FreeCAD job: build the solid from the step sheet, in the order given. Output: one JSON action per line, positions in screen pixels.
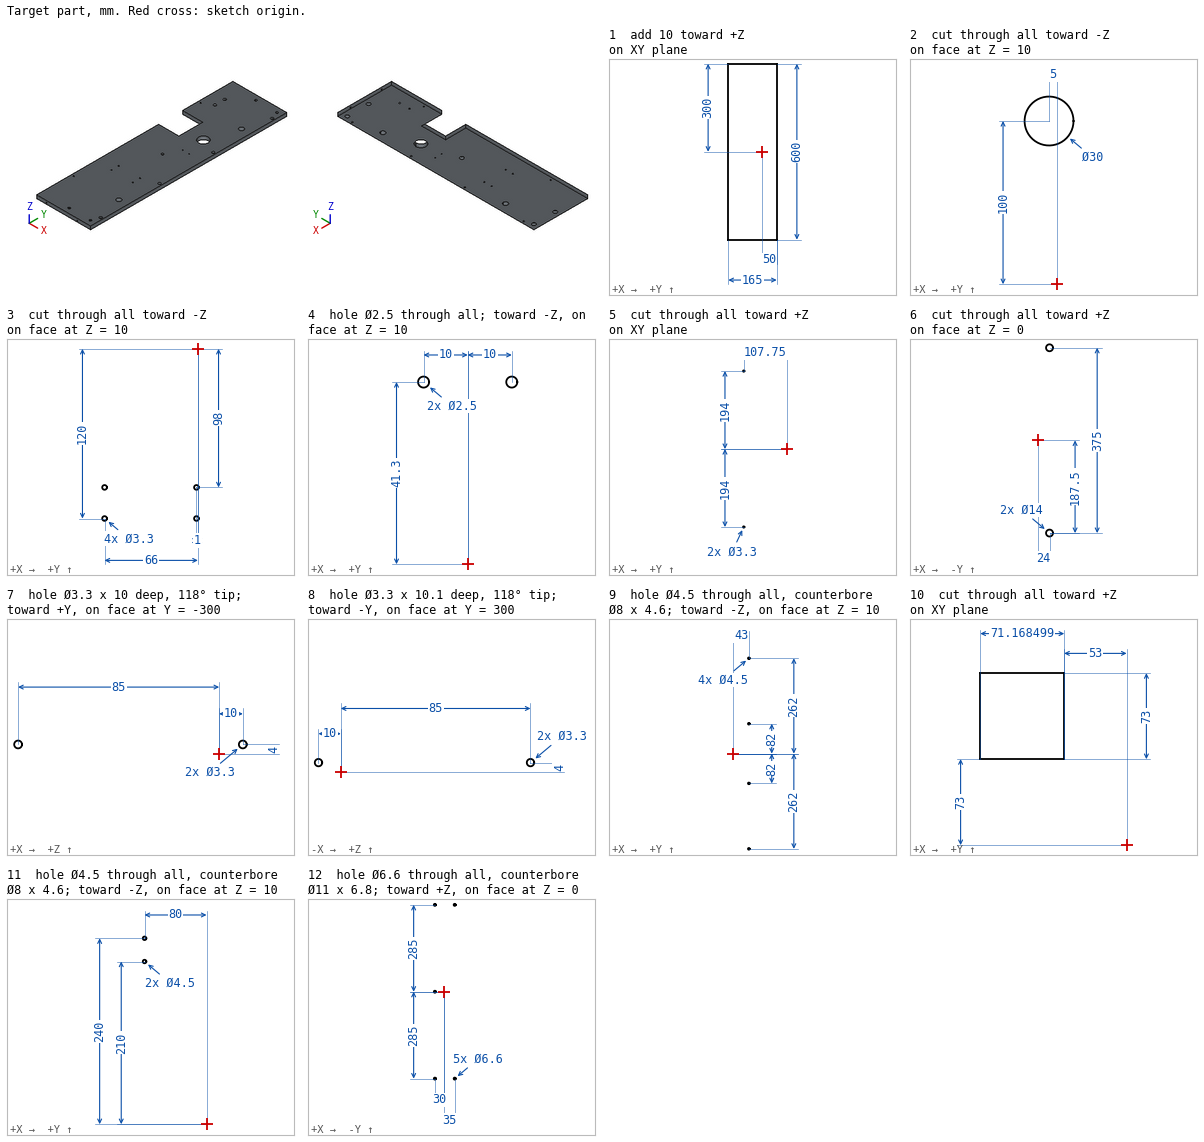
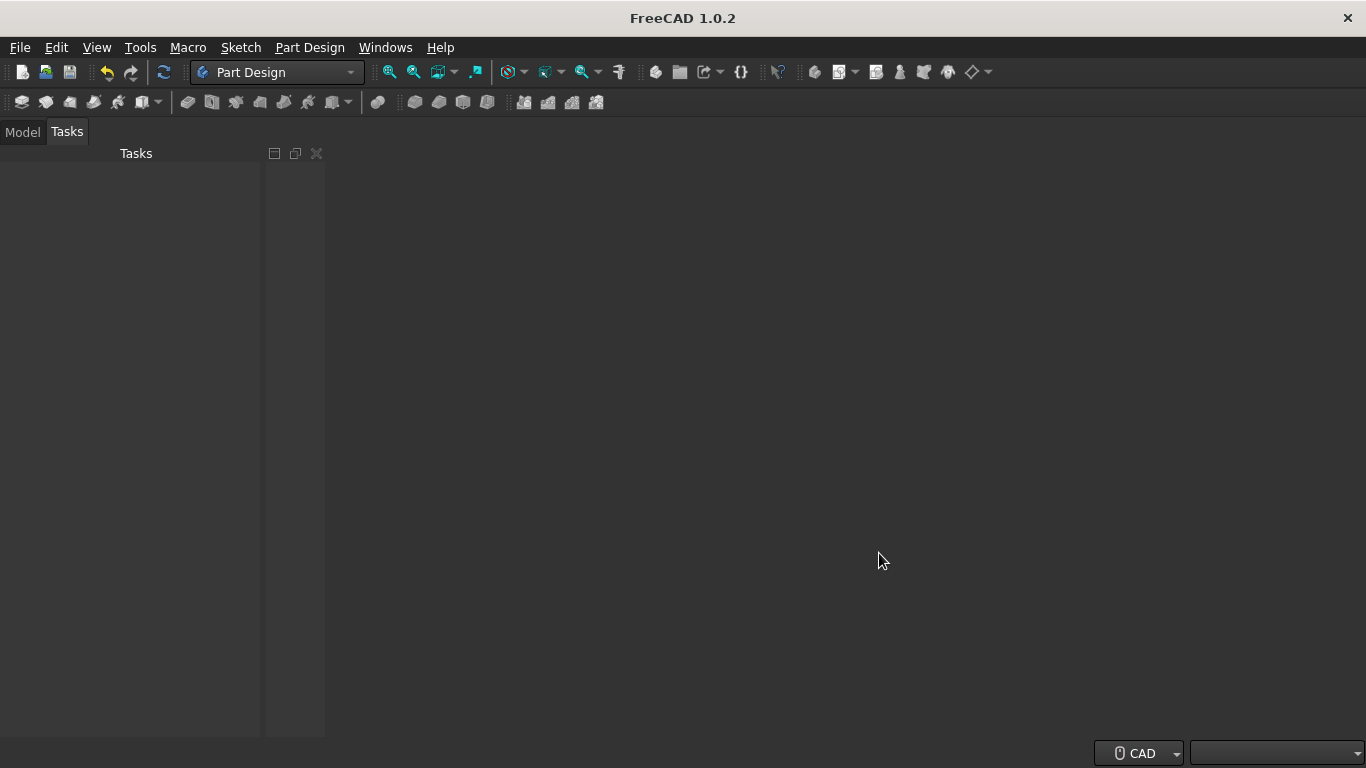
{"action": "key", "text": "ctrl+n"}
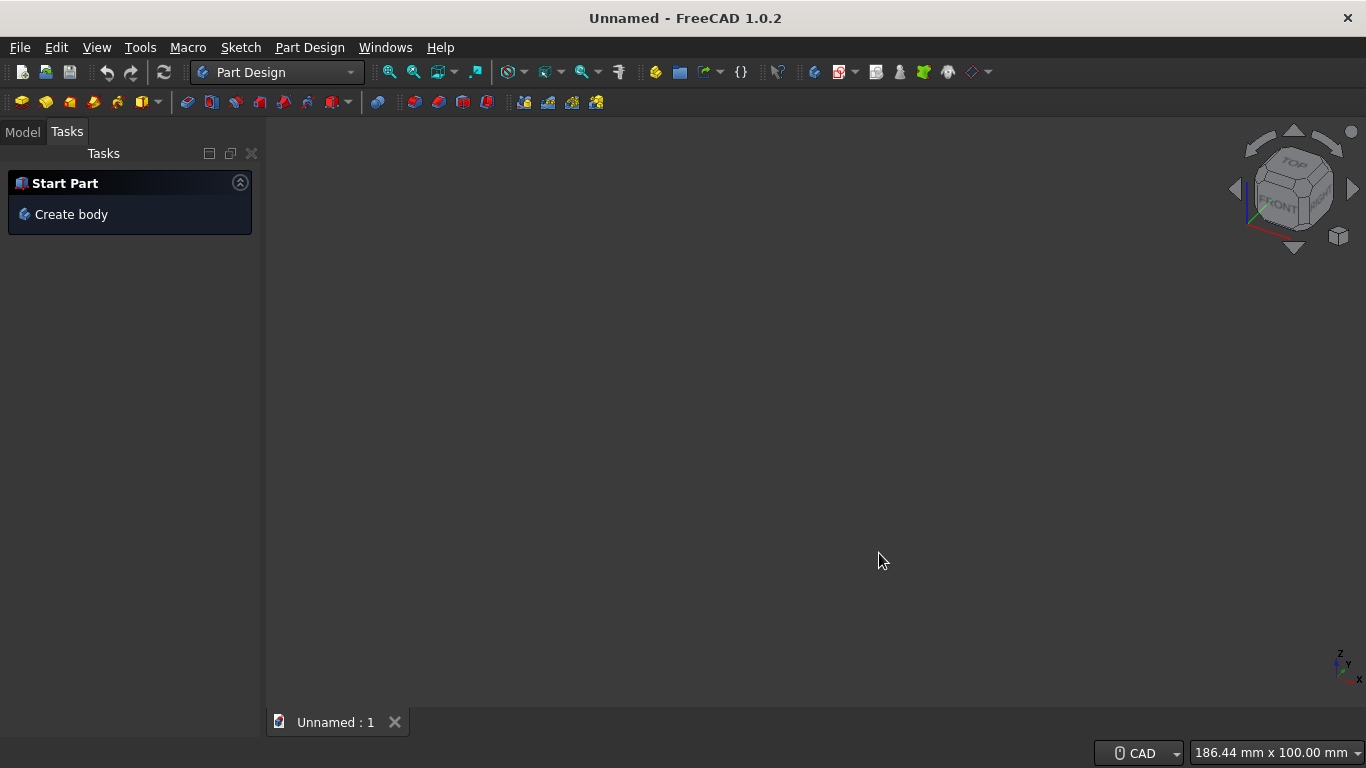
{"action": "left_click", "coordinate": [840, 72]}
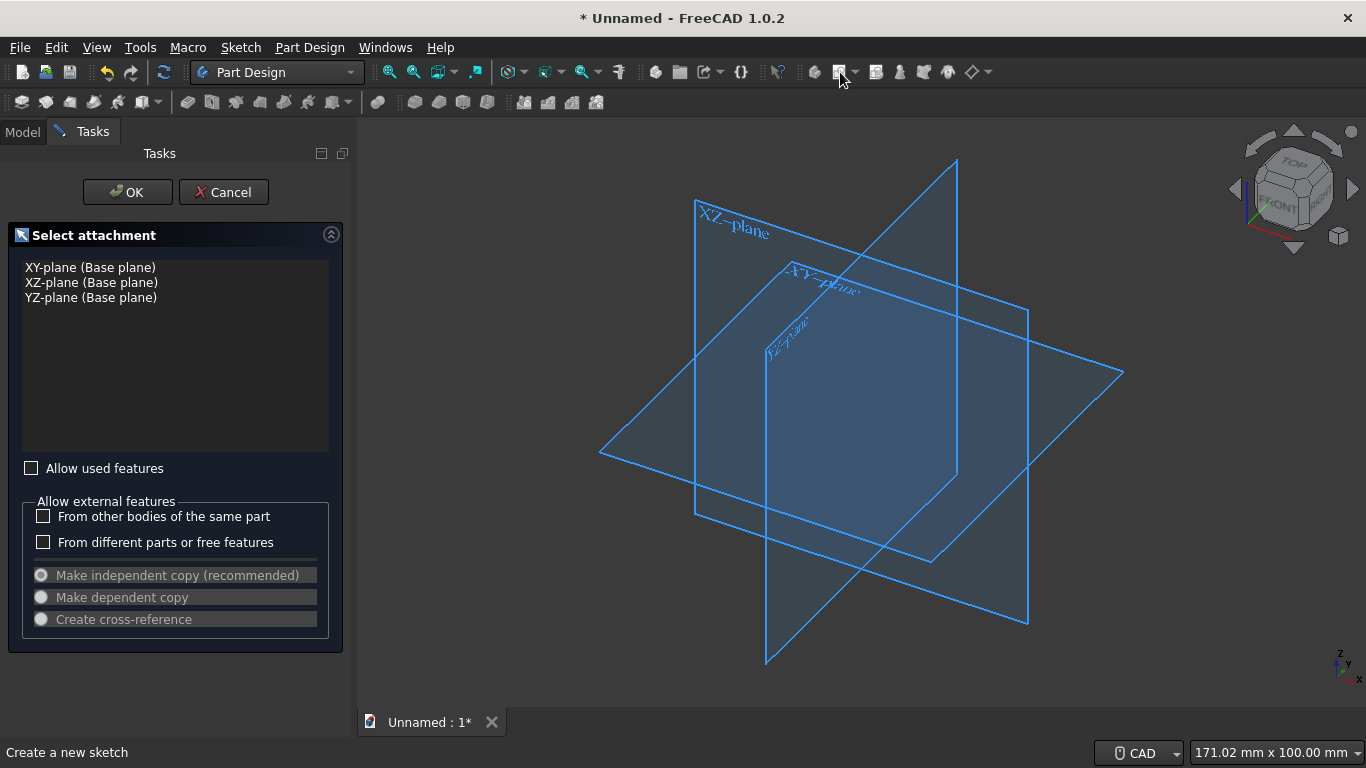
{"action": "left_click", "coordinate": [82, 268]}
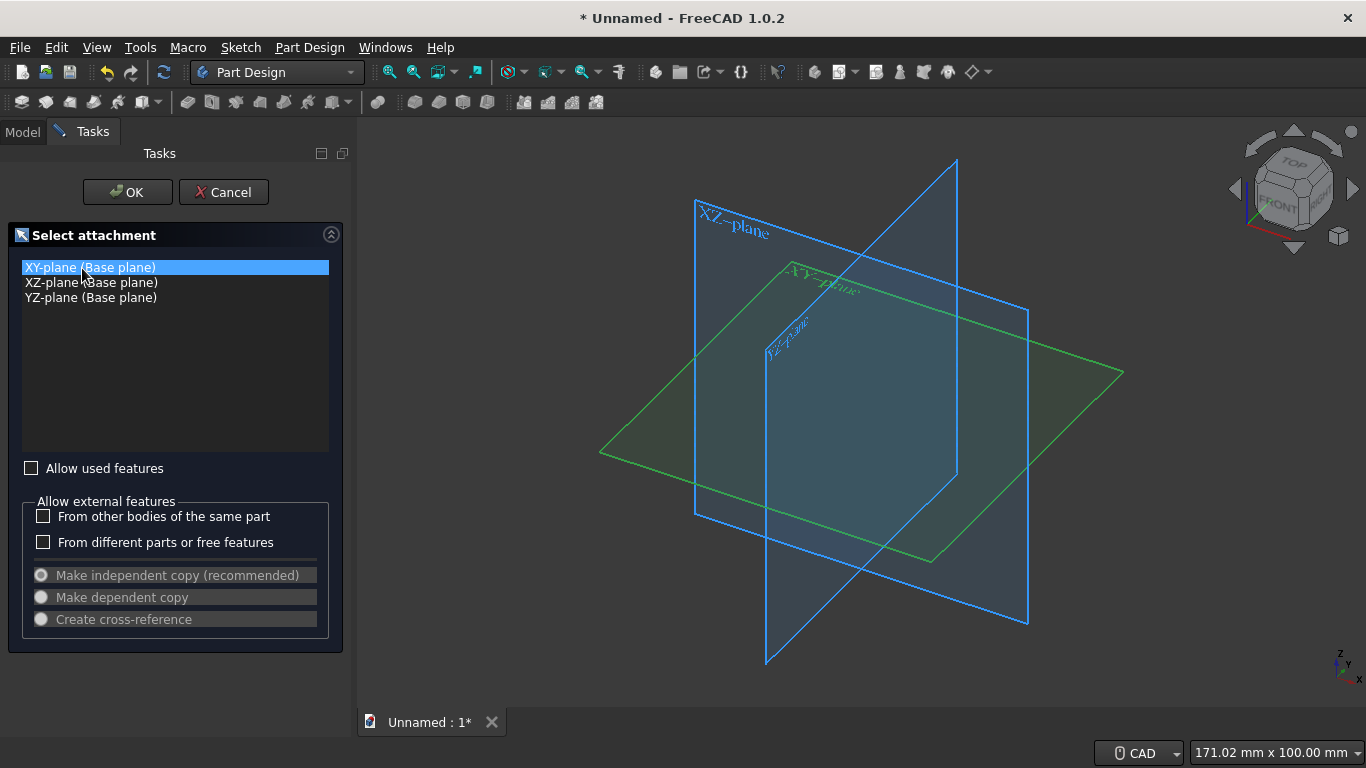
{"action": "left_click", "coordinate": [128, 192]}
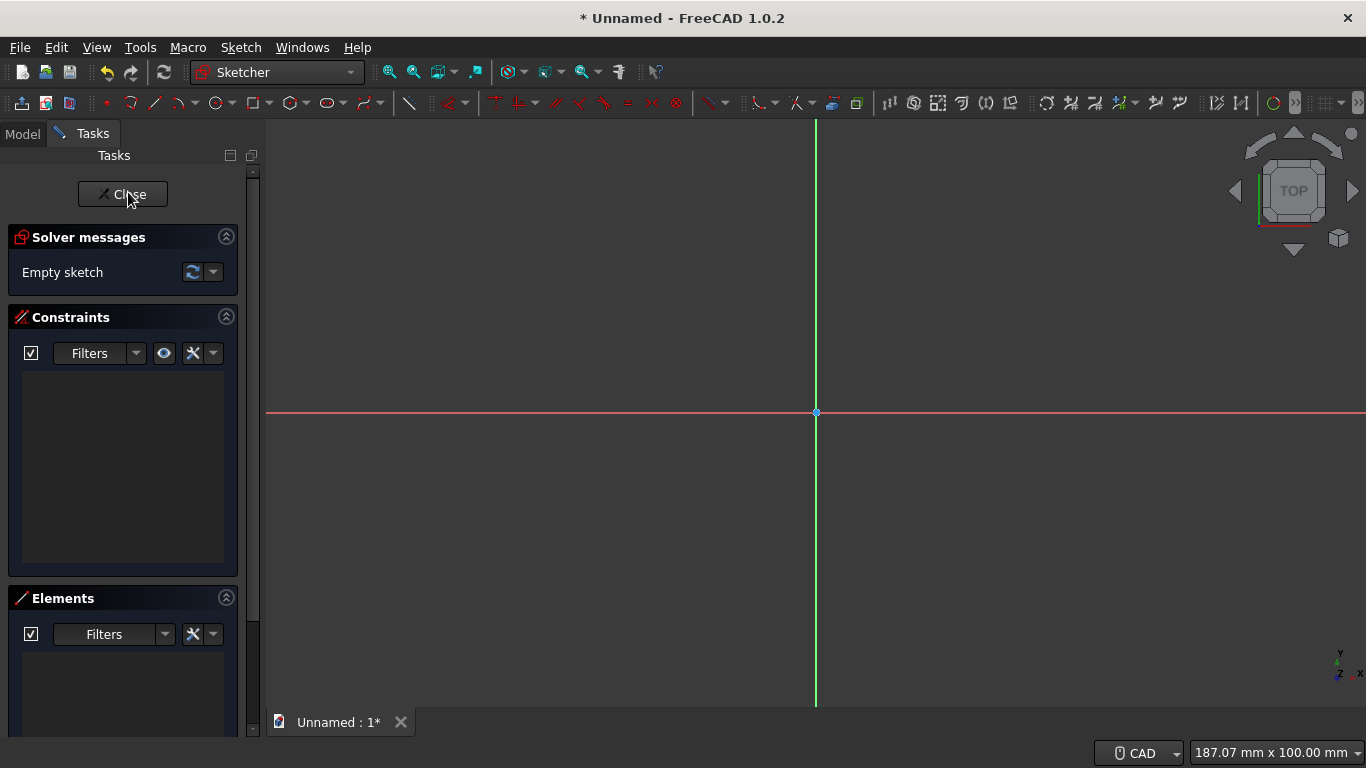
{"action": "scroll", "coordinate": [763, 413], "scroll_direction": "down", "scroll_amount": 11}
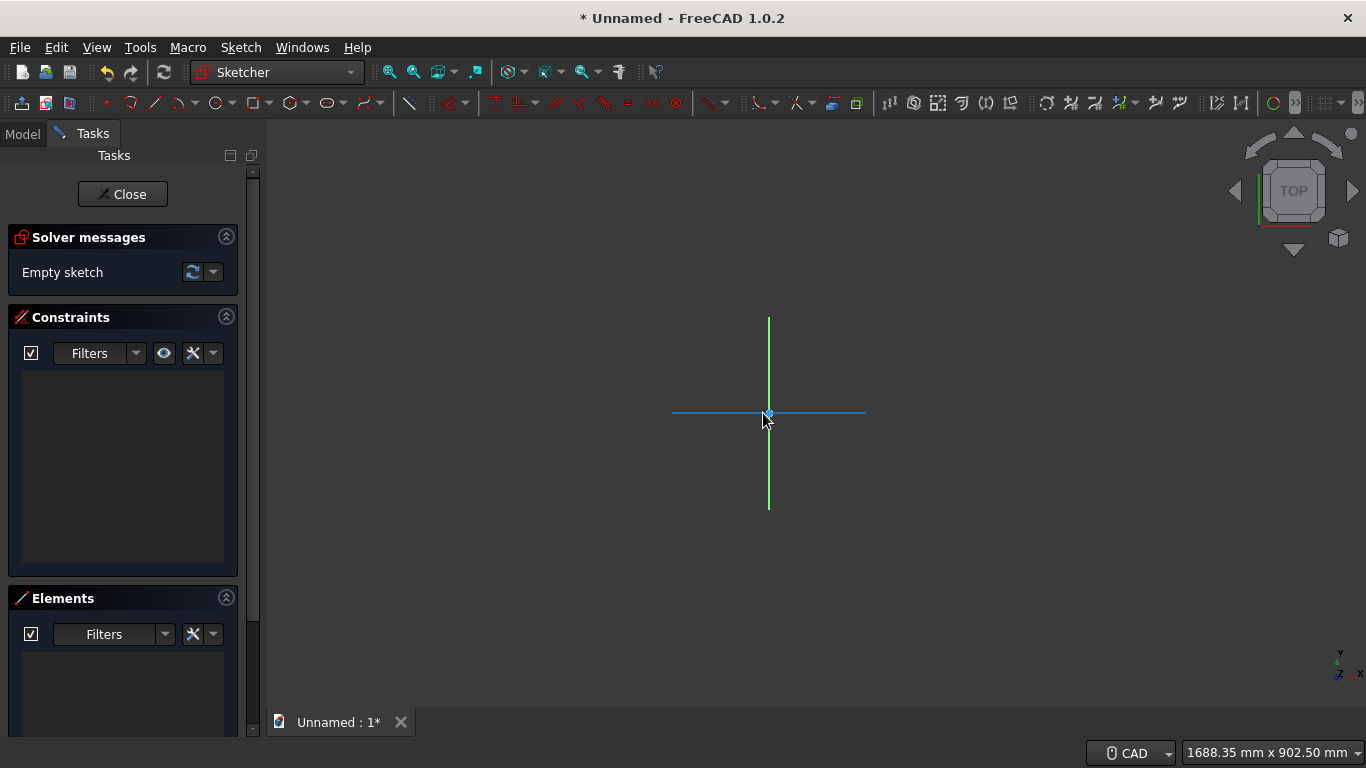
{"action": "left_click", "coordinate": [254, 104]}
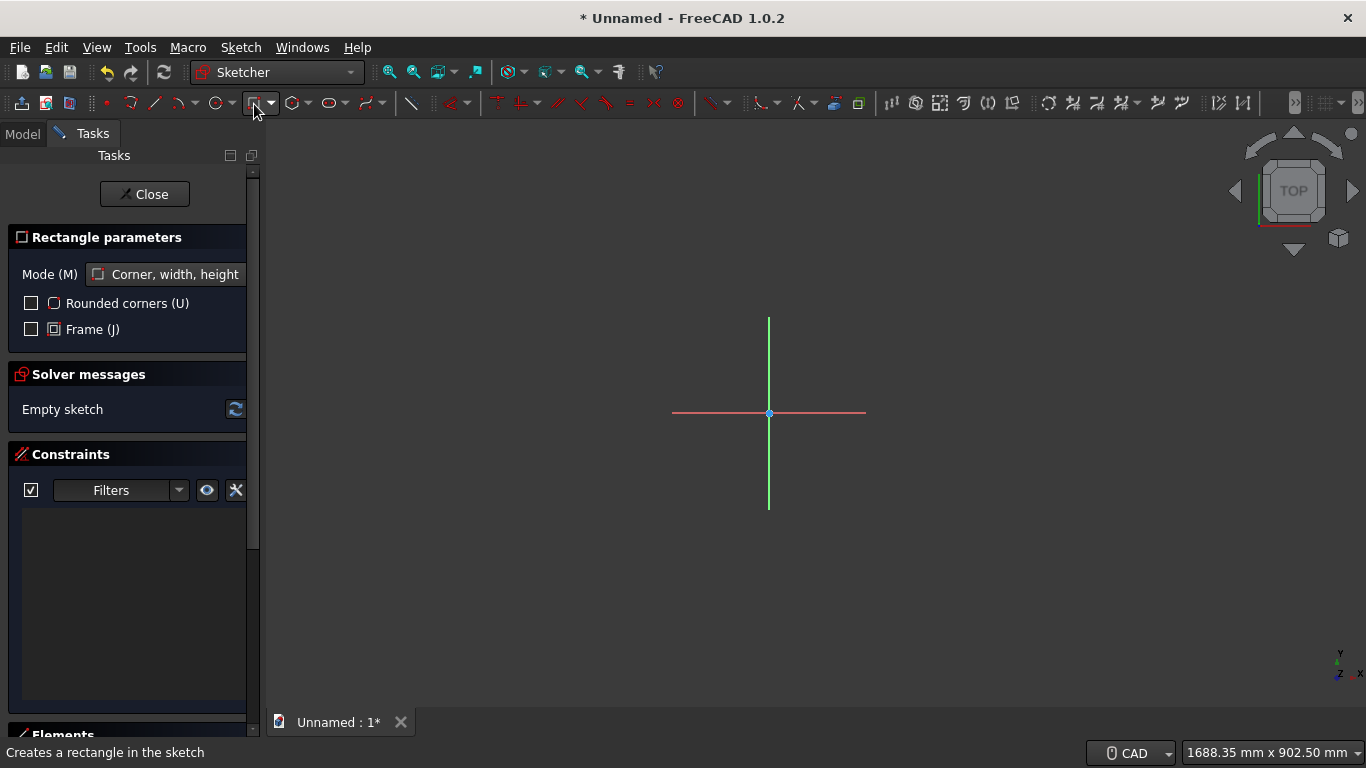
{"action": "left_click", "coordinate": [694, 218]}
{"action": "mouse_move", "coordinate": [802, 609]}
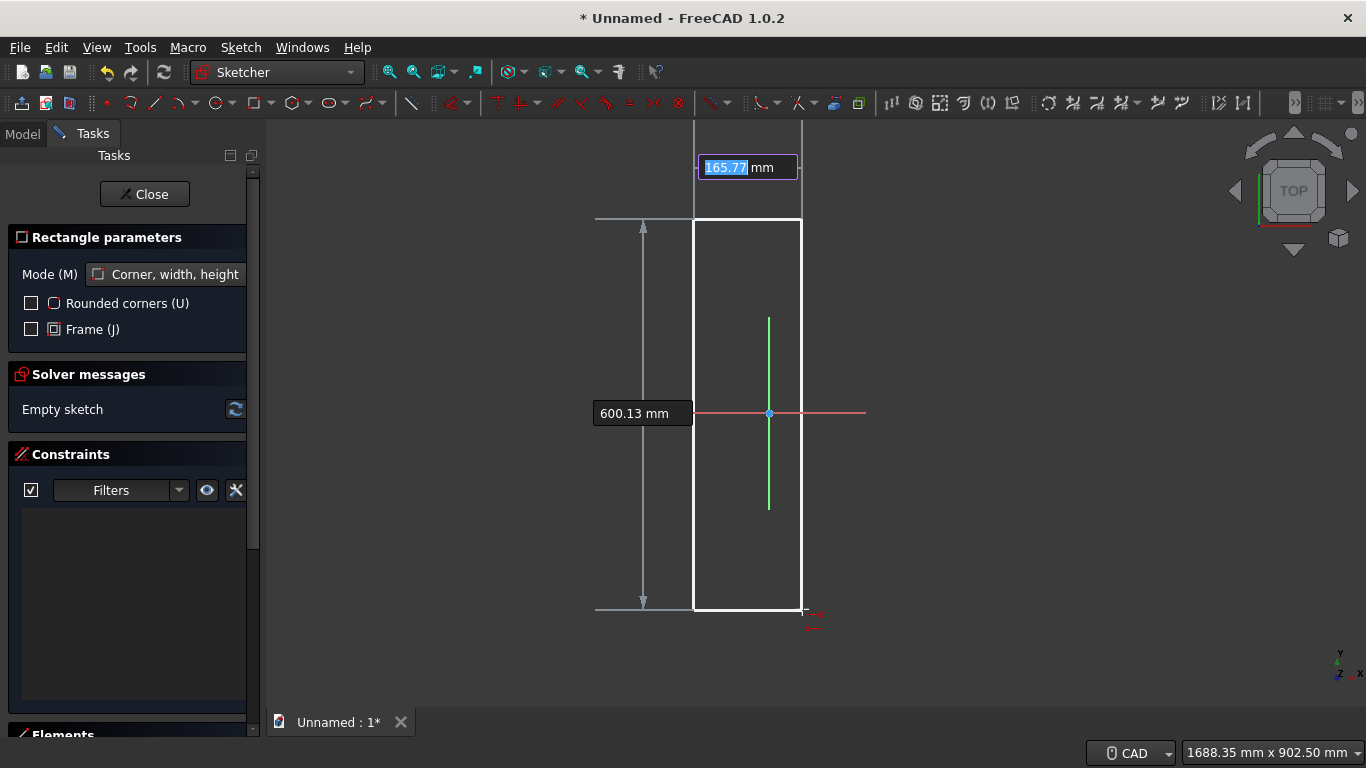
{"action": "type", "text": "165"}
{"action": "key", "text": "Tab"}
{"action": "type", "text": "600"}
{"action": "key", "text": "Return"}
{"action": "key", "text": "Escape"}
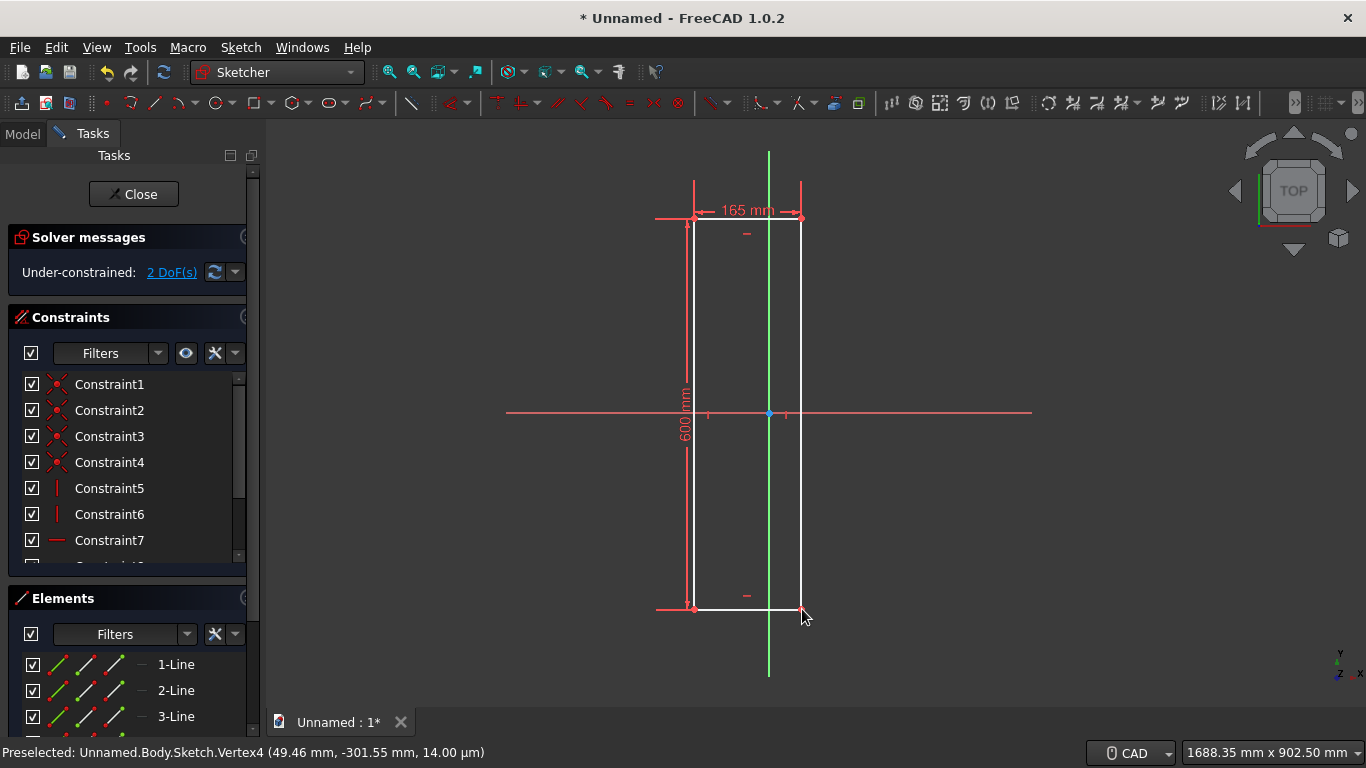
{"action": "left_click", "coordinate": [450, 104]}